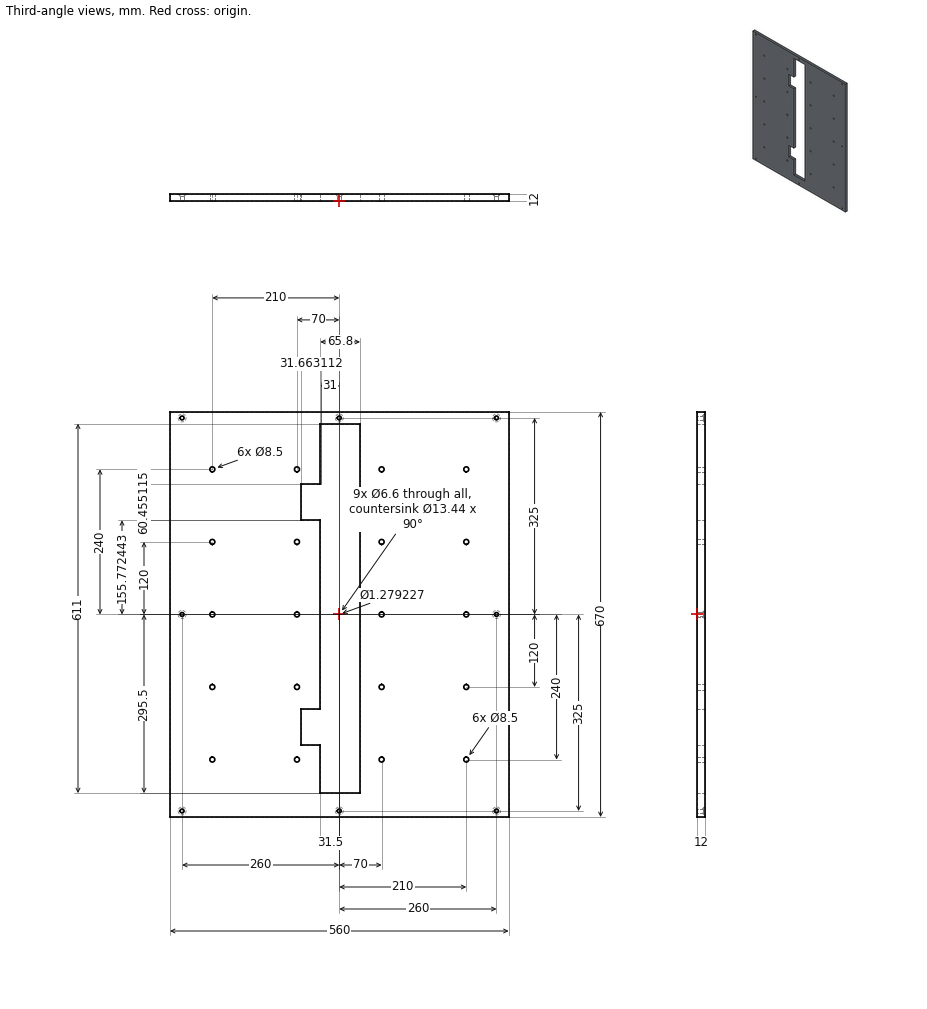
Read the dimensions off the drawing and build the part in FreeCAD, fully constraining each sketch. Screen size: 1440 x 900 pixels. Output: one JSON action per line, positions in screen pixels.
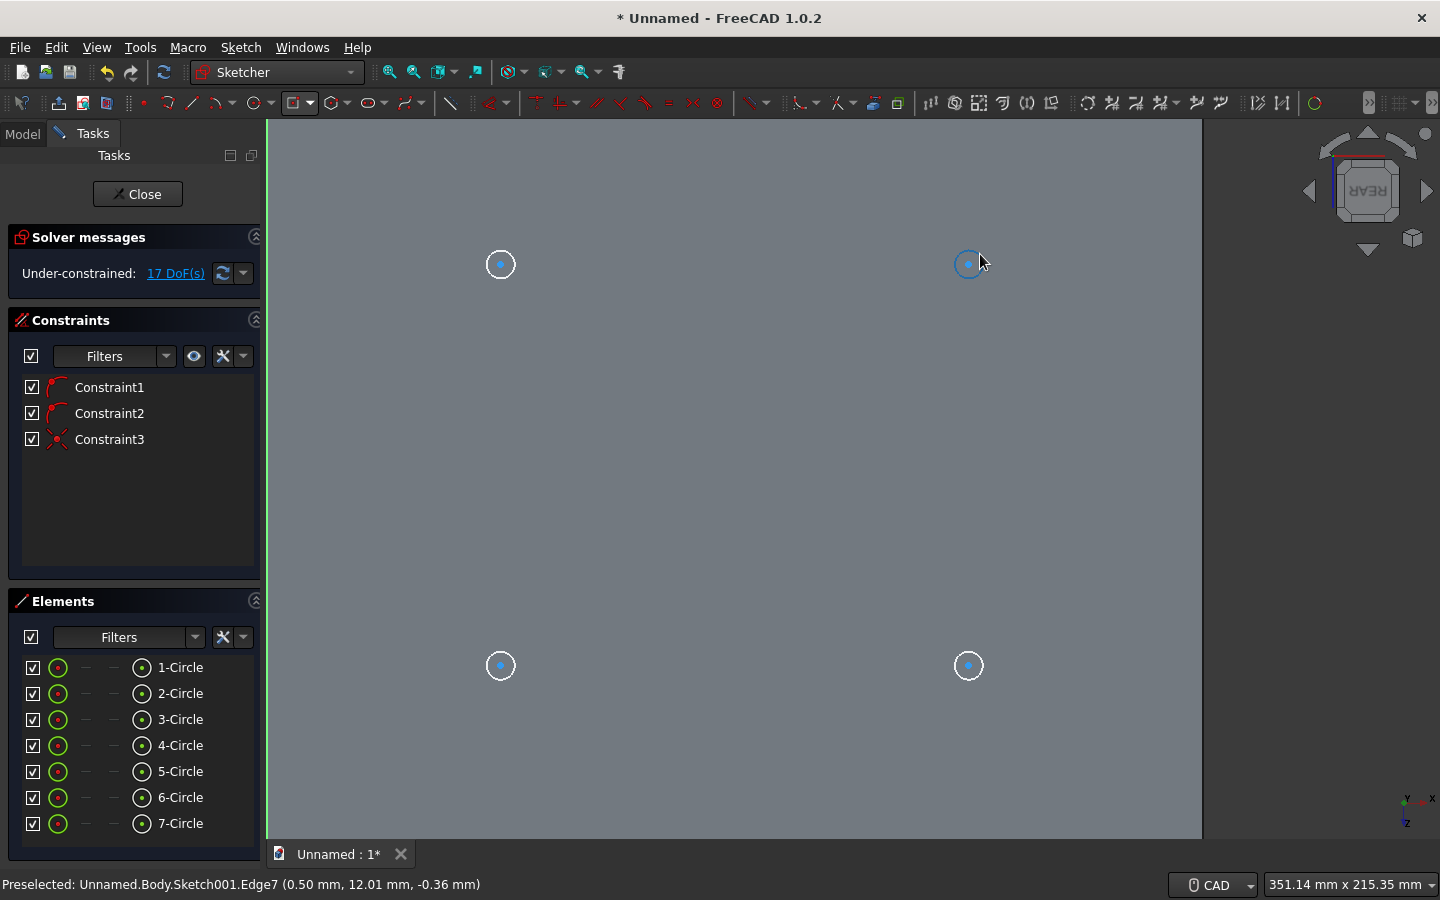
{"action": "left_click", "coordinate": [979, 255]}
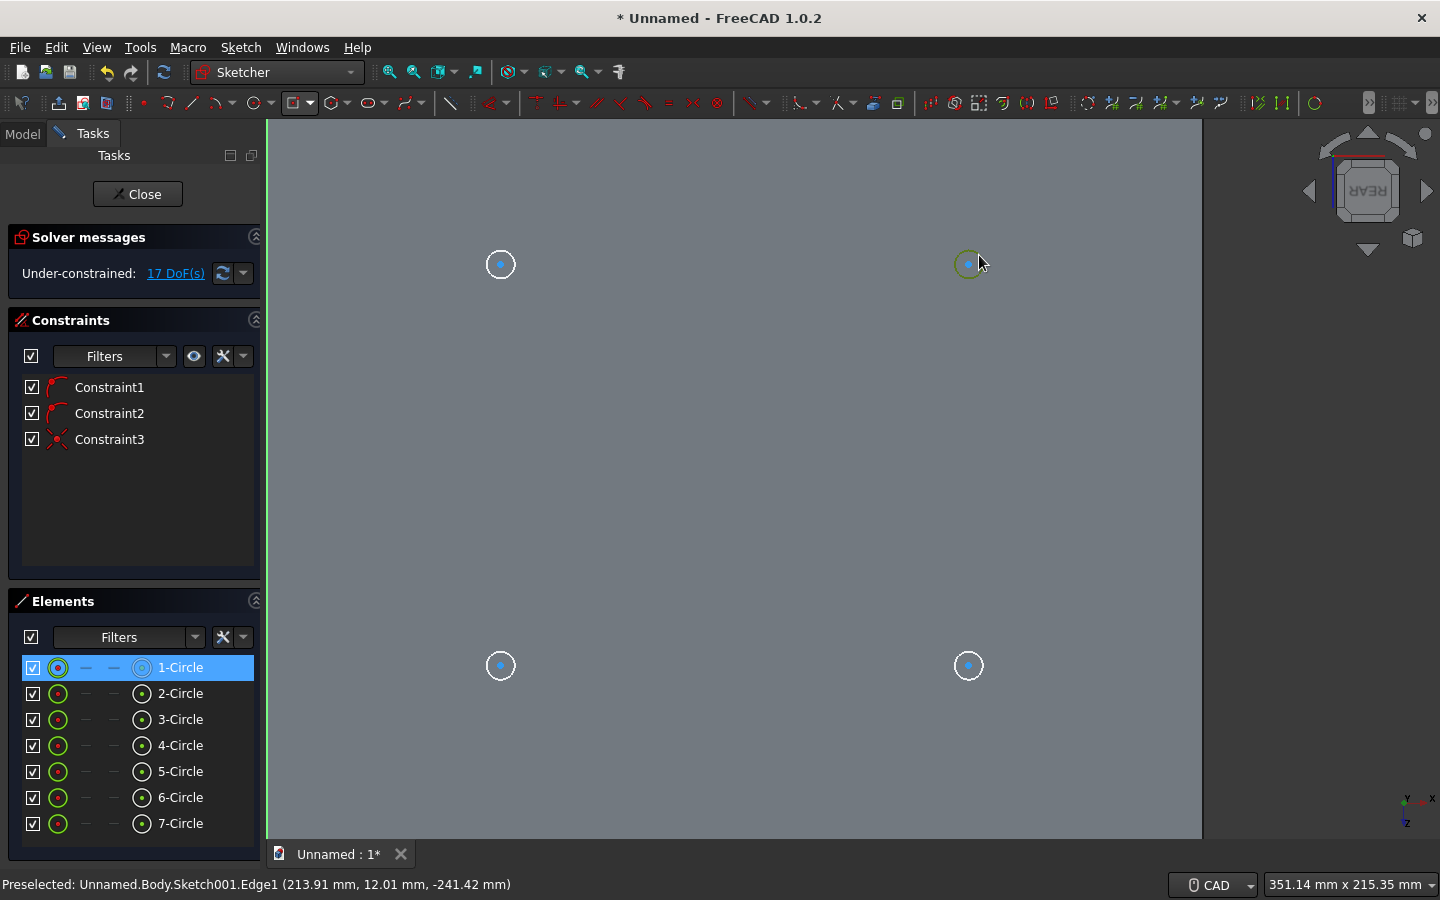
{"action": "left_click", "coordinate": [511, 255]}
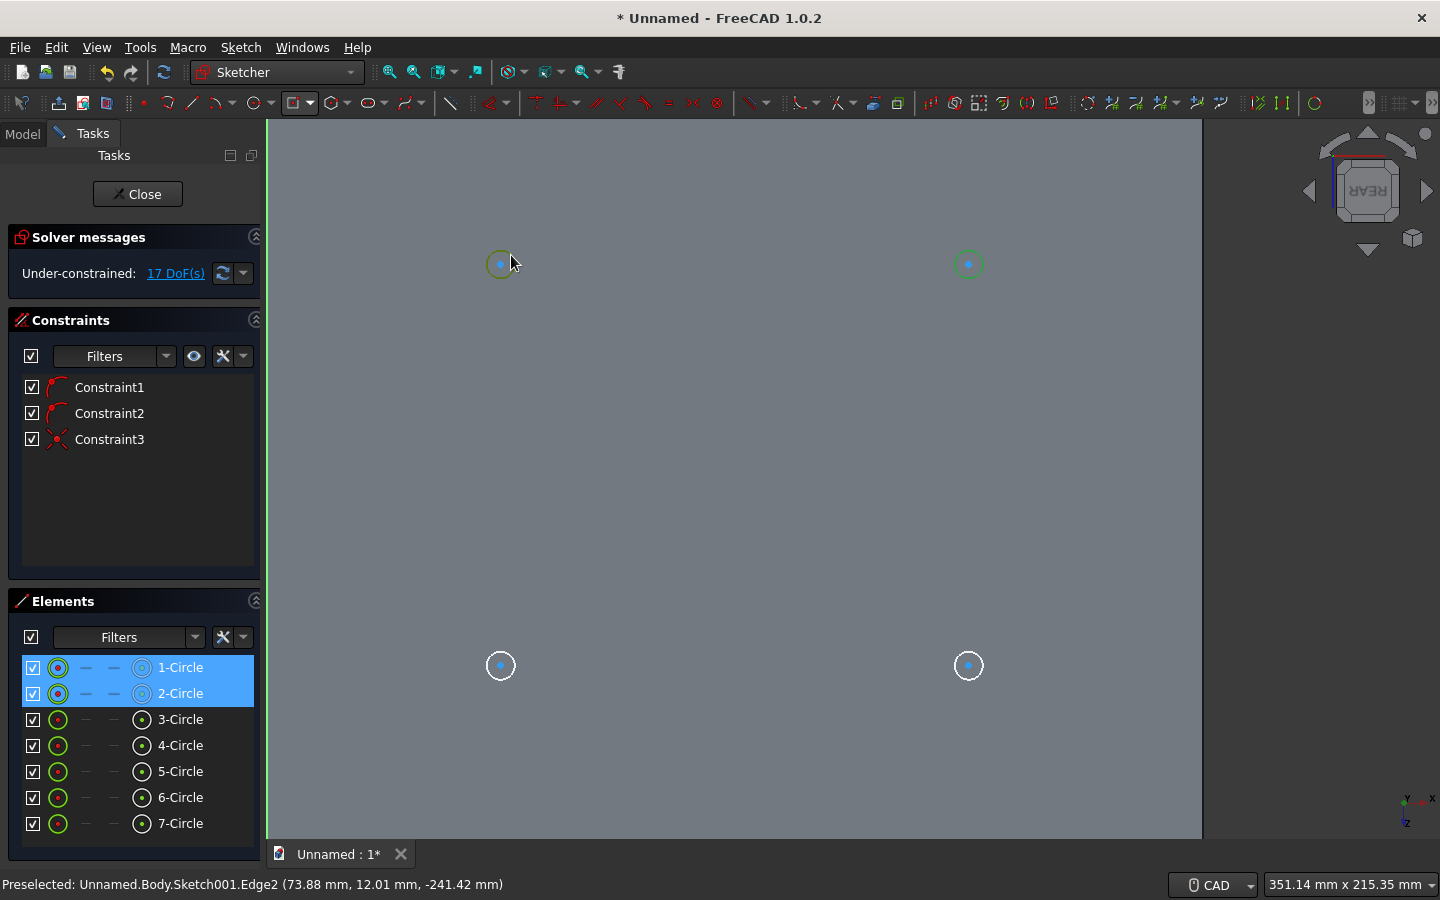
{"action": "left_click", "coordinate": [979, 656]}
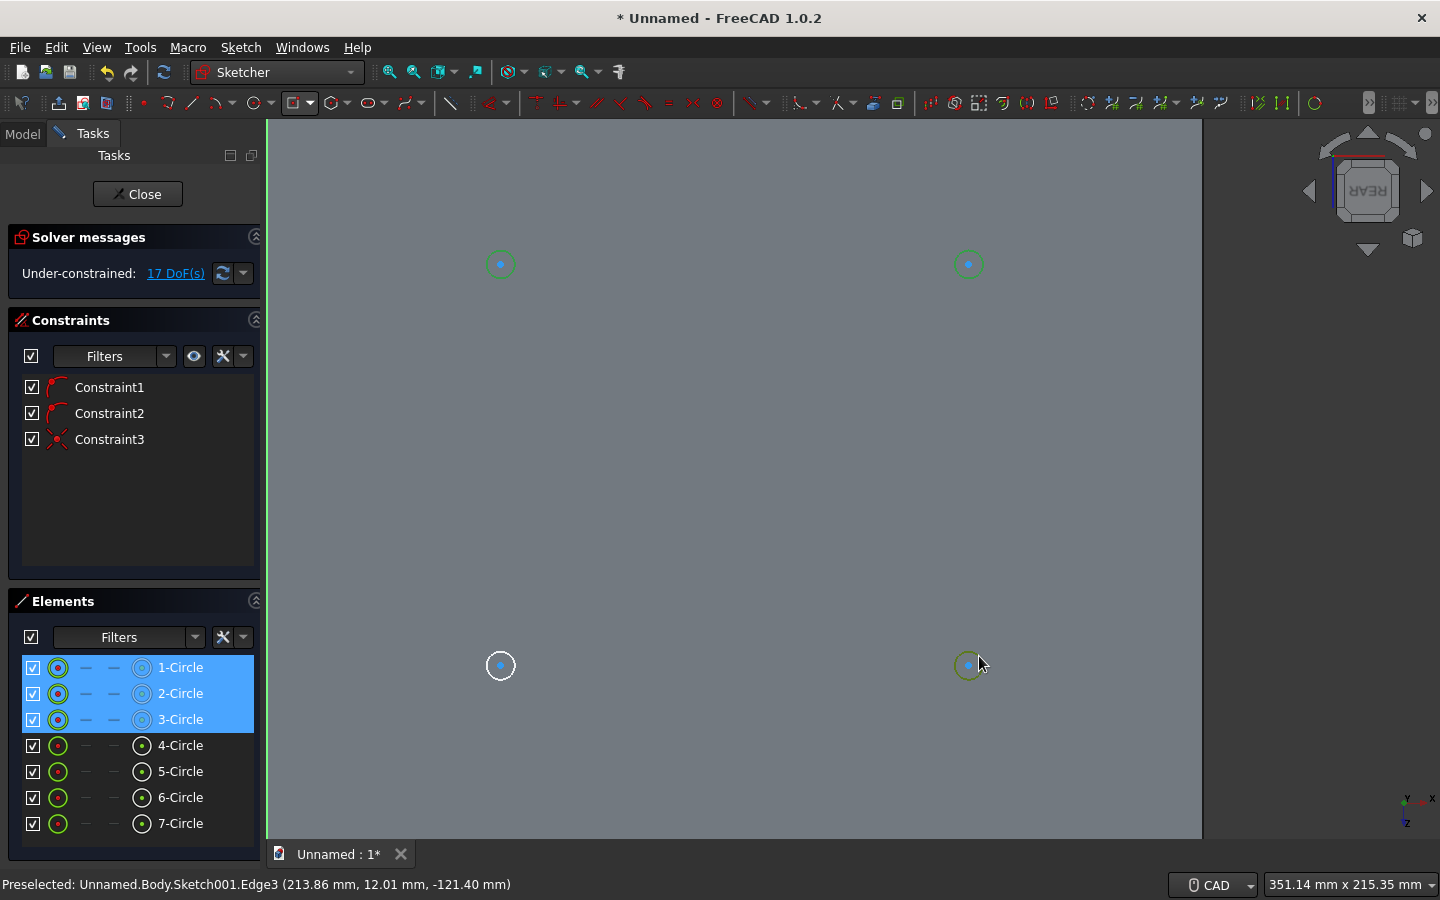
{"action": "left_click", "coordinate": [511, 656]}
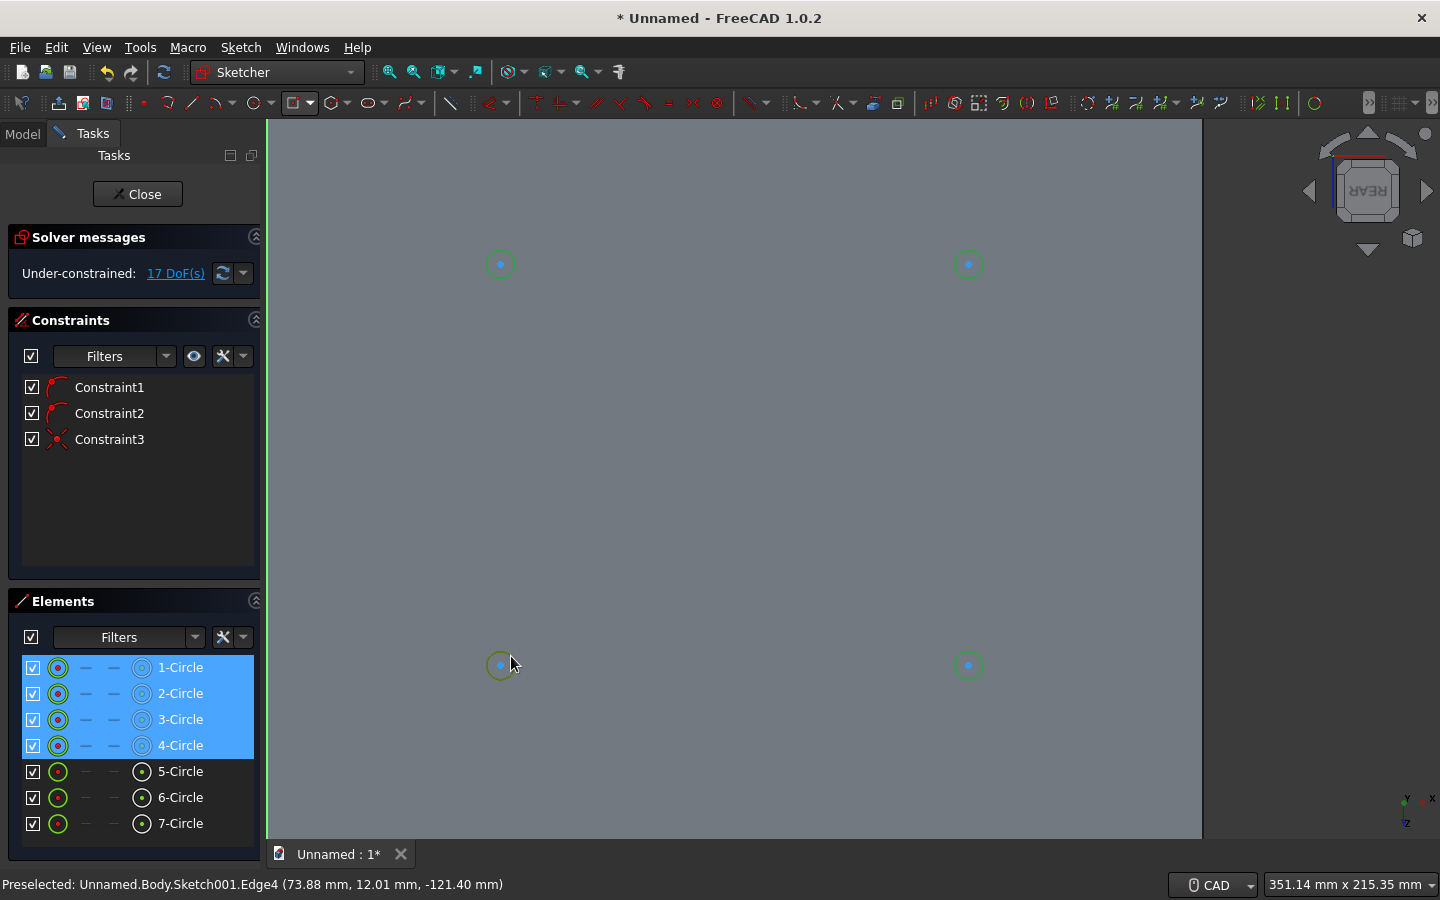
{"action": "scroll", "coordinate": [980, 252], "scroll_direction": "down", "scroll_amount": 3}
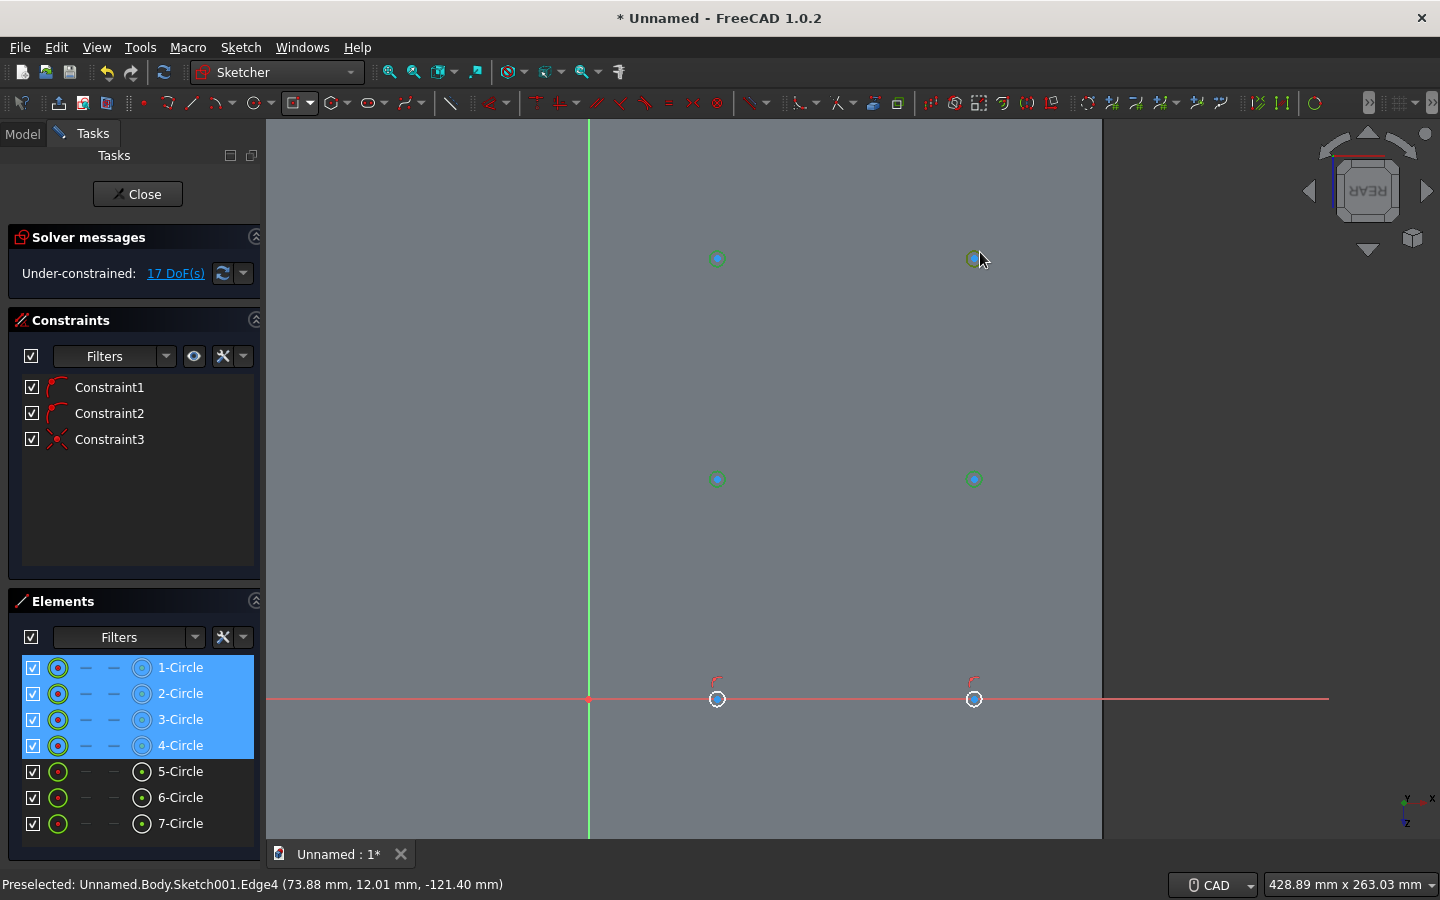
{"action": "scroll", "coordinate": [723, 694], "scroll_direction": "up", "scroll_amount": 5}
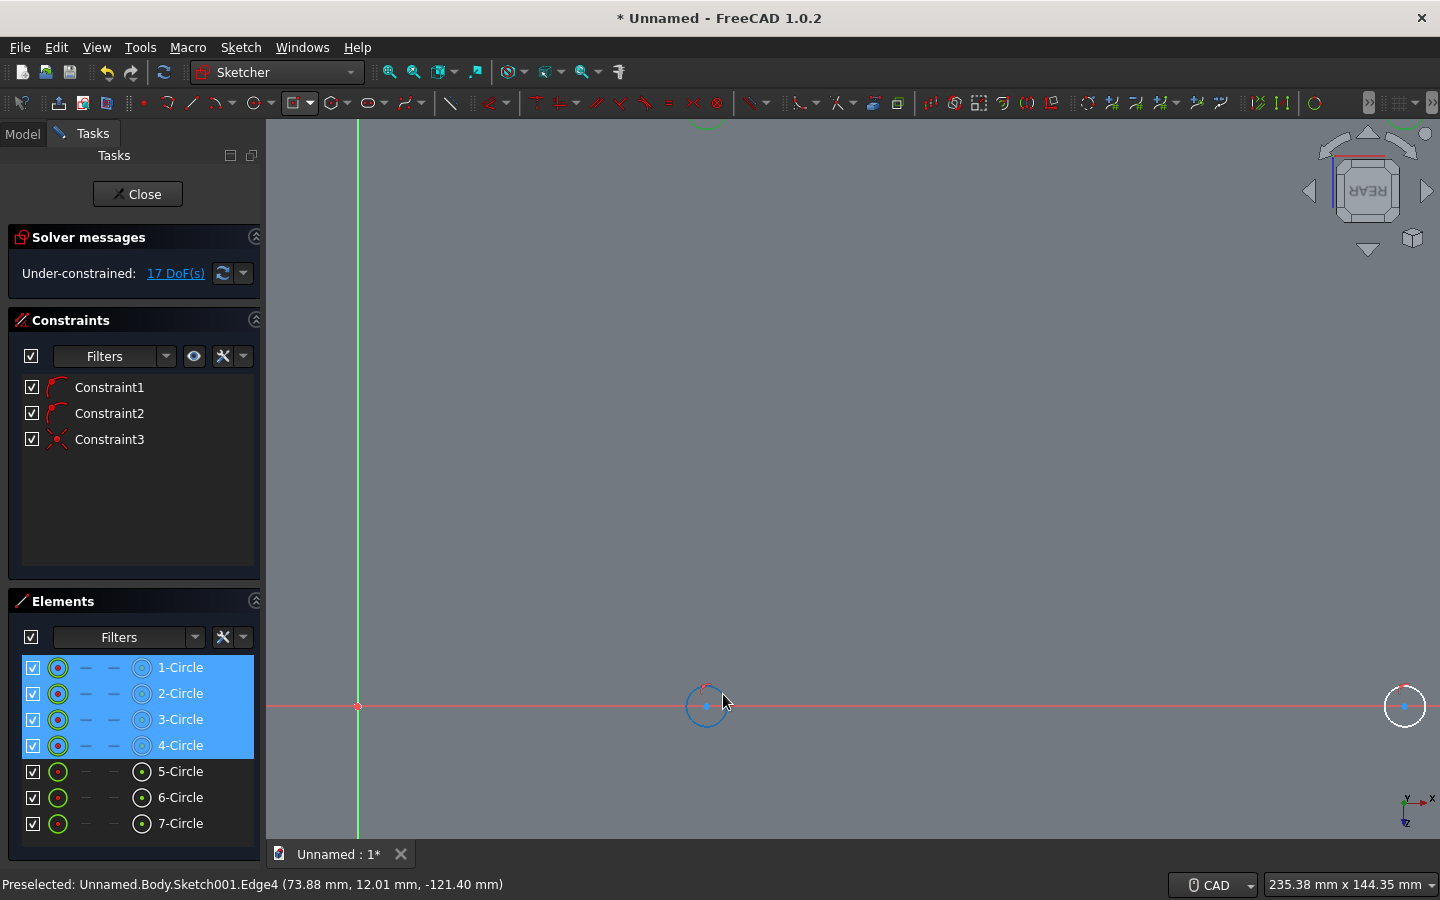
{"action": "left_click", "coordinate": [721, 692]}